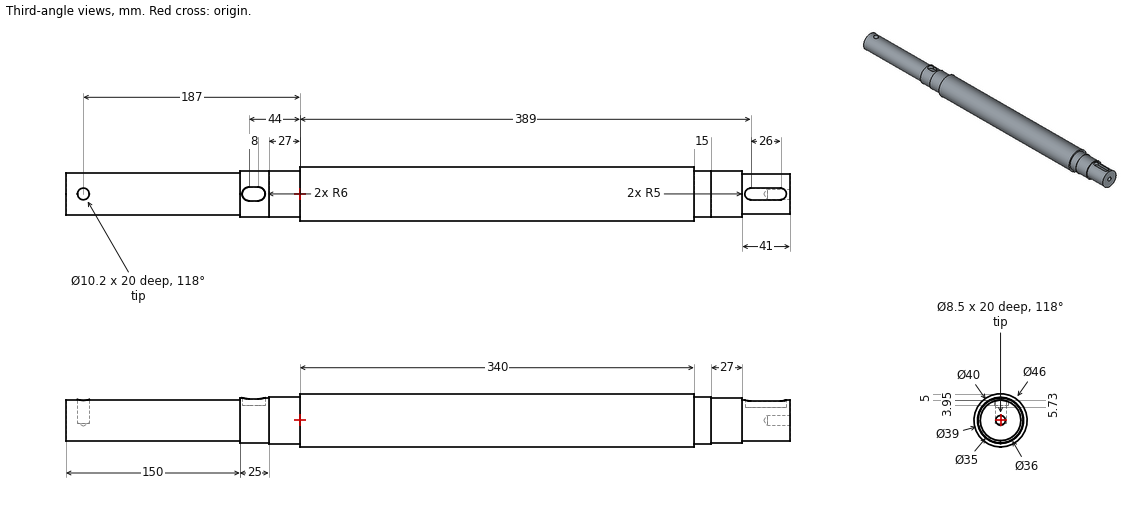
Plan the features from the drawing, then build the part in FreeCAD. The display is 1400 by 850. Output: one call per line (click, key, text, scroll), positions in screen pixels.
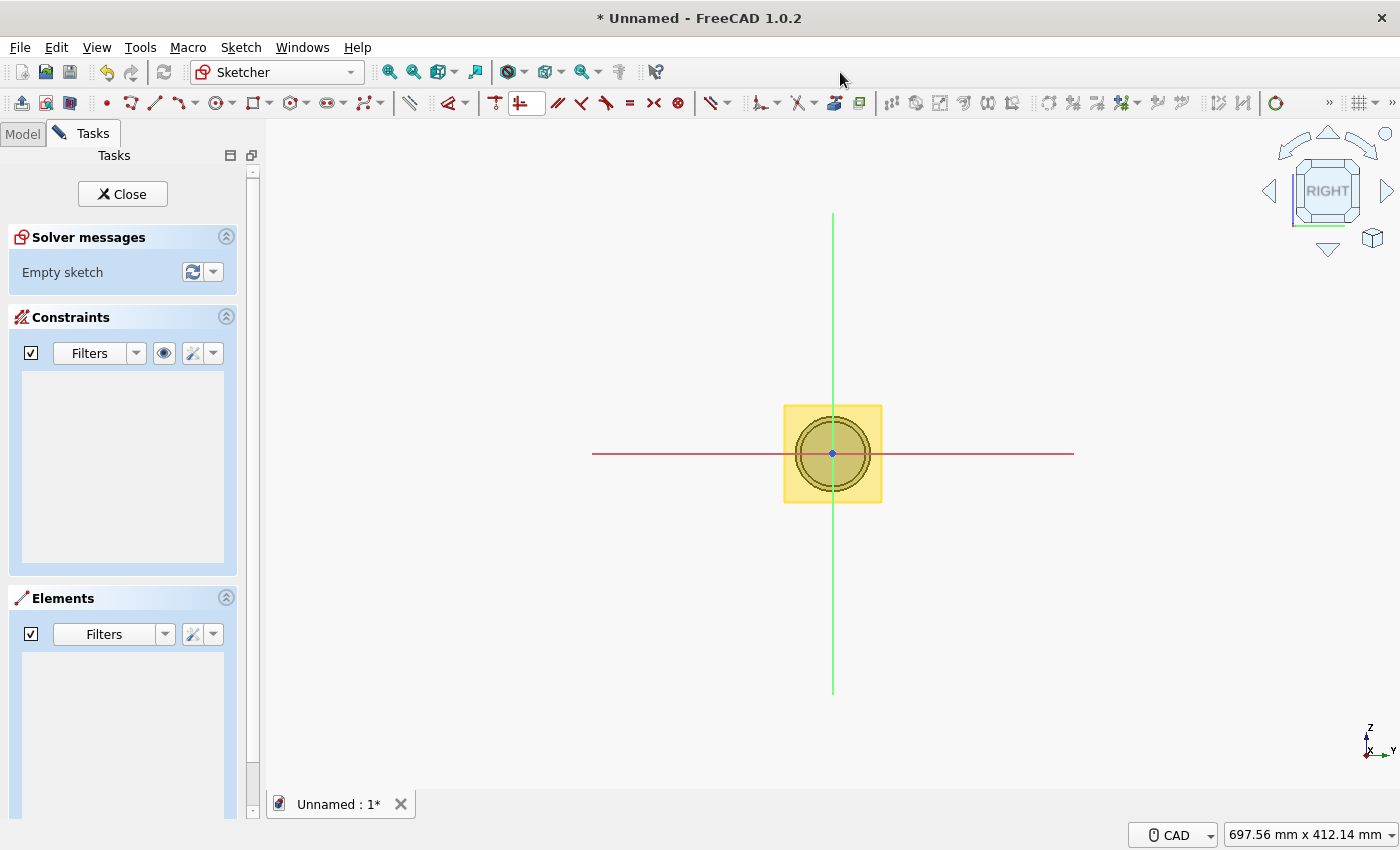
scroll(844, 454, up, 10)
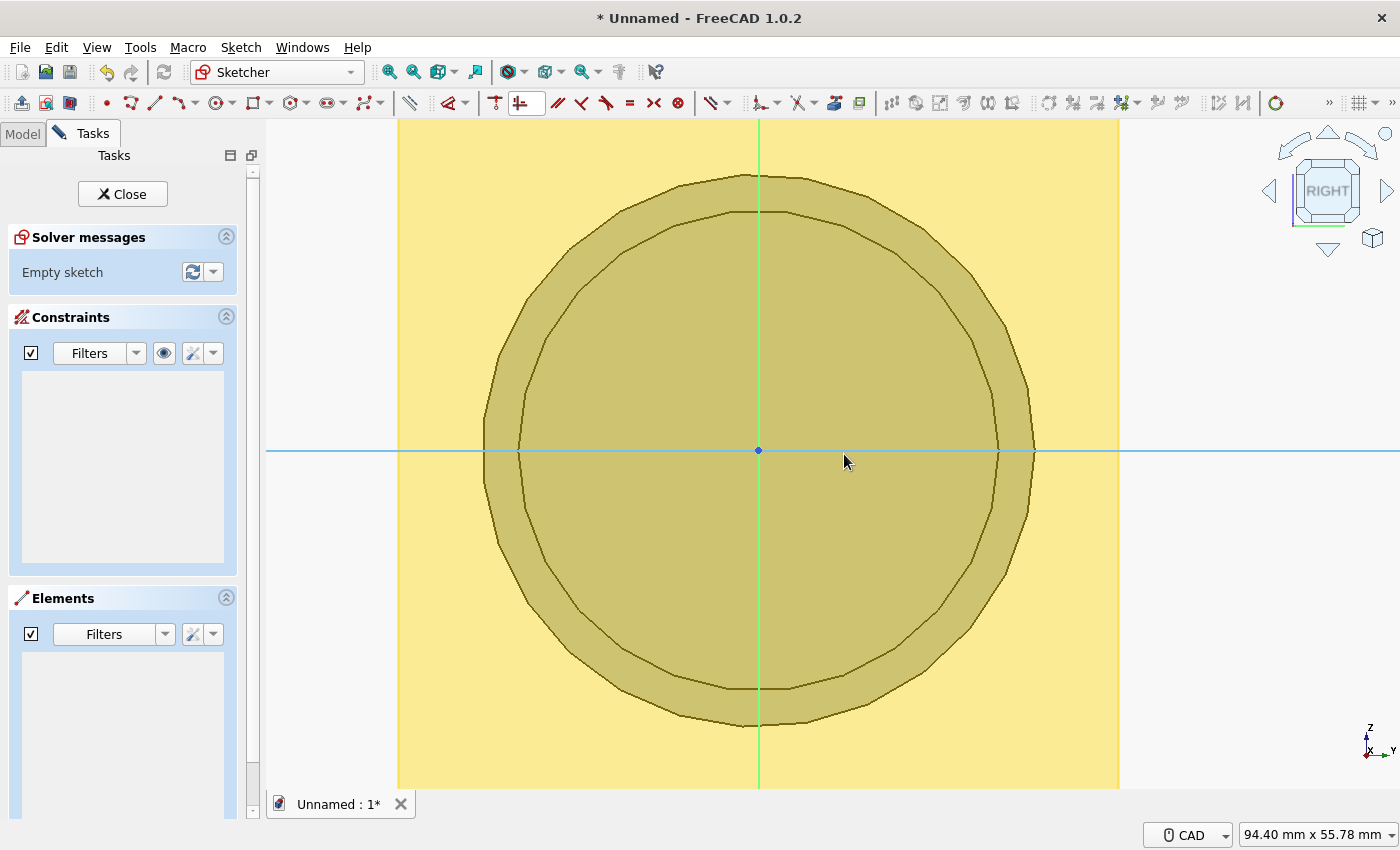
click(216, 104)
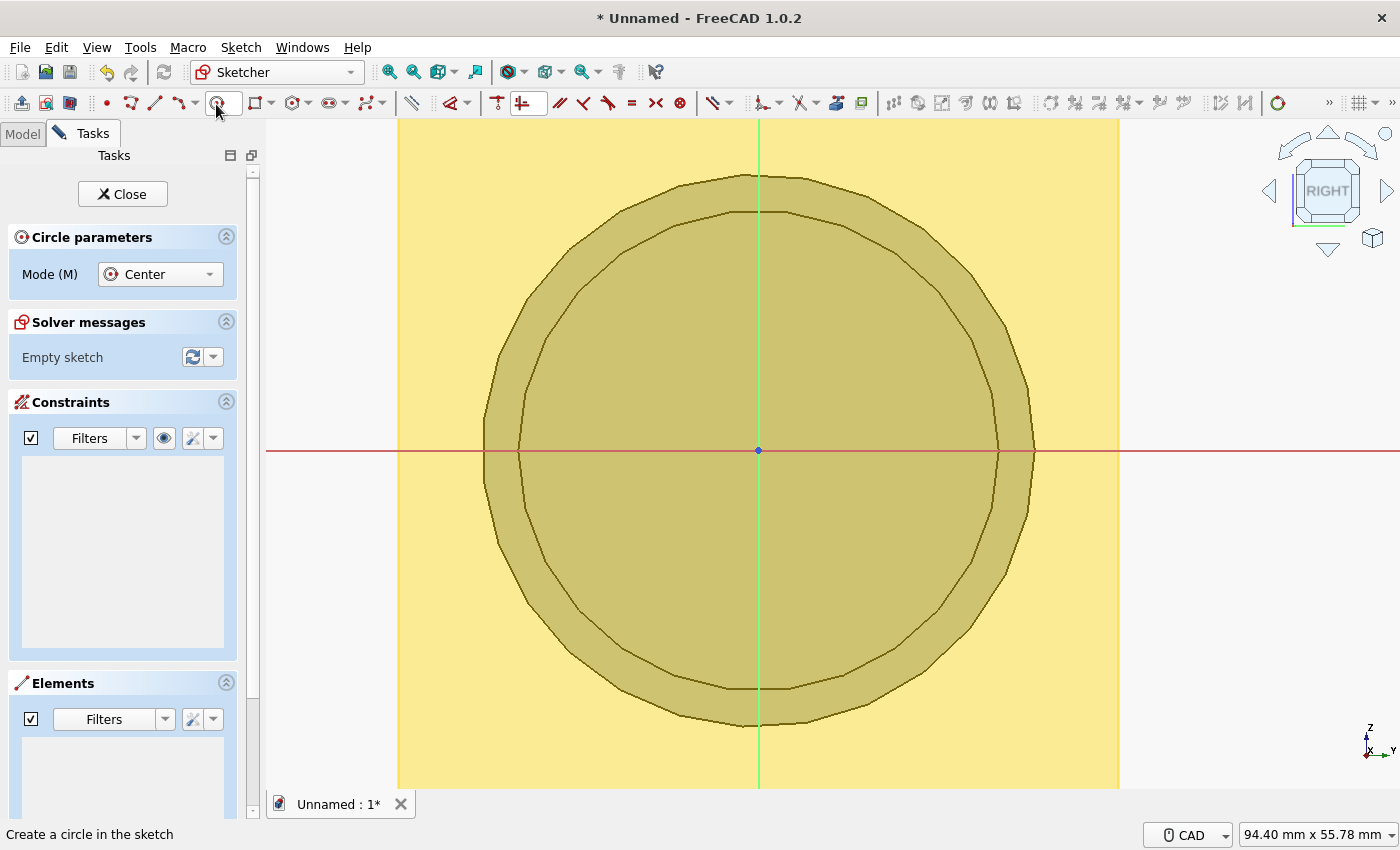
click(759, 451)
click(924, 285)
key(Escape)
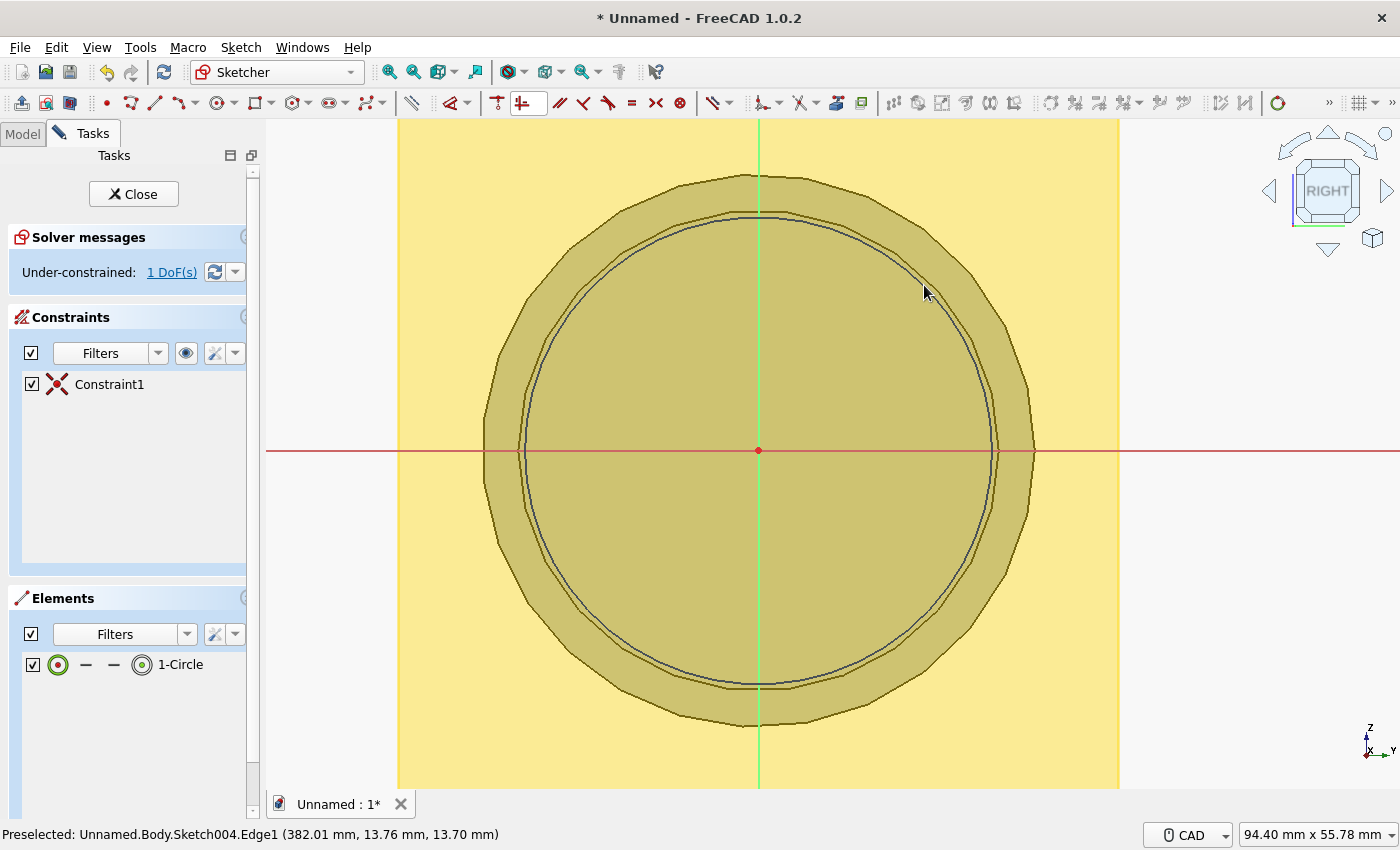
key(d)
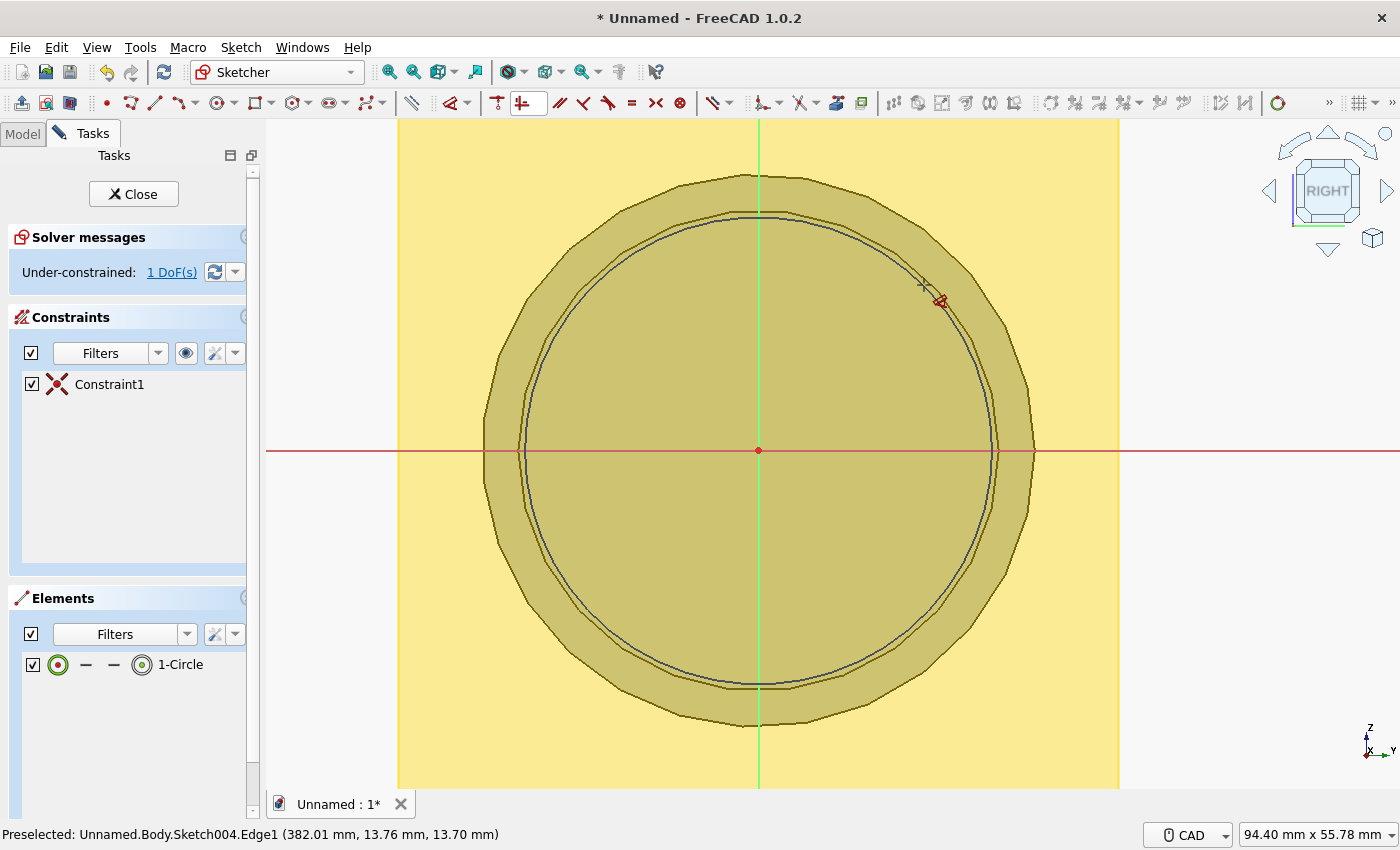
click(923, 285)
click(946, 262)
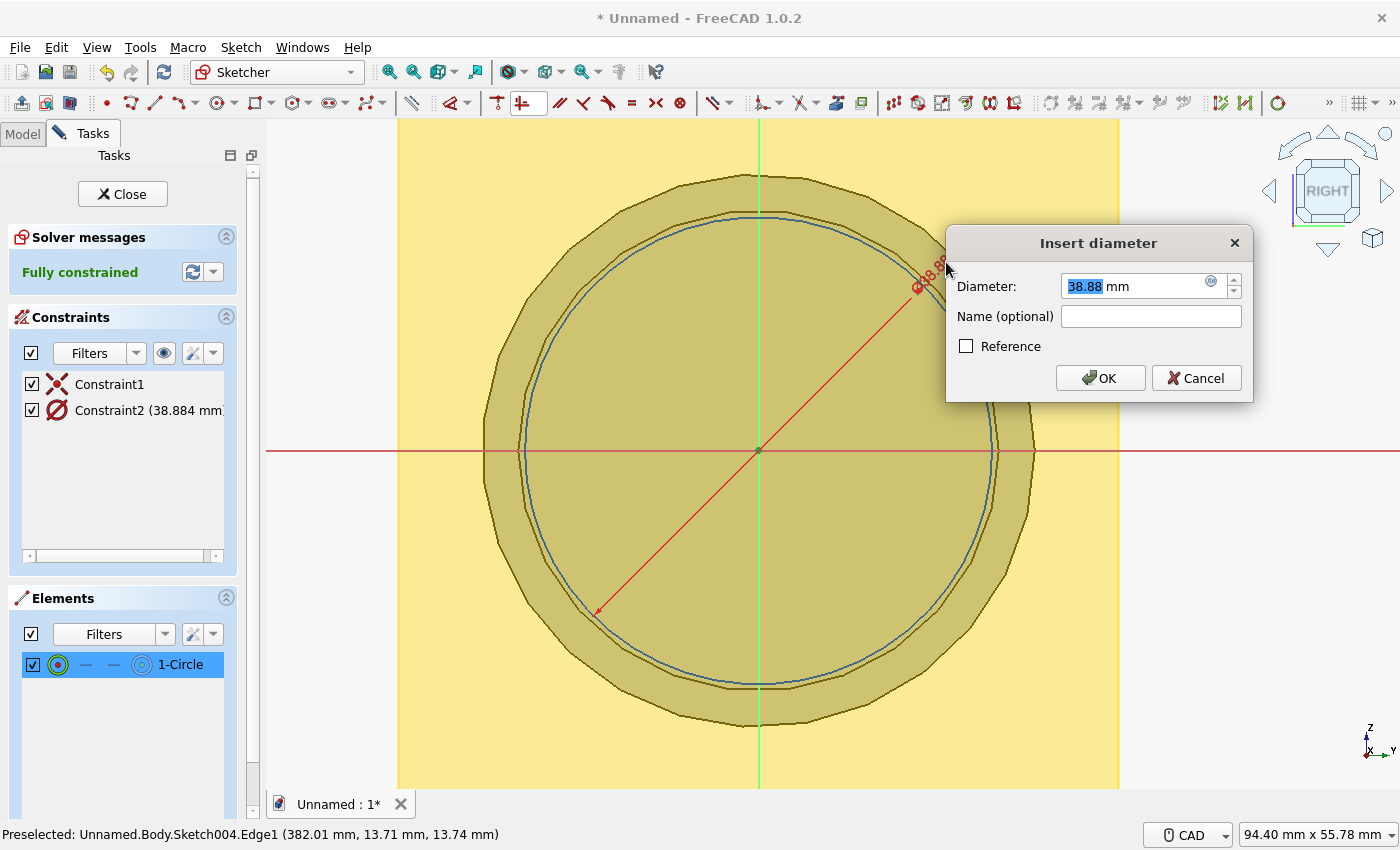
text(39)
key(Return)
key(Escape)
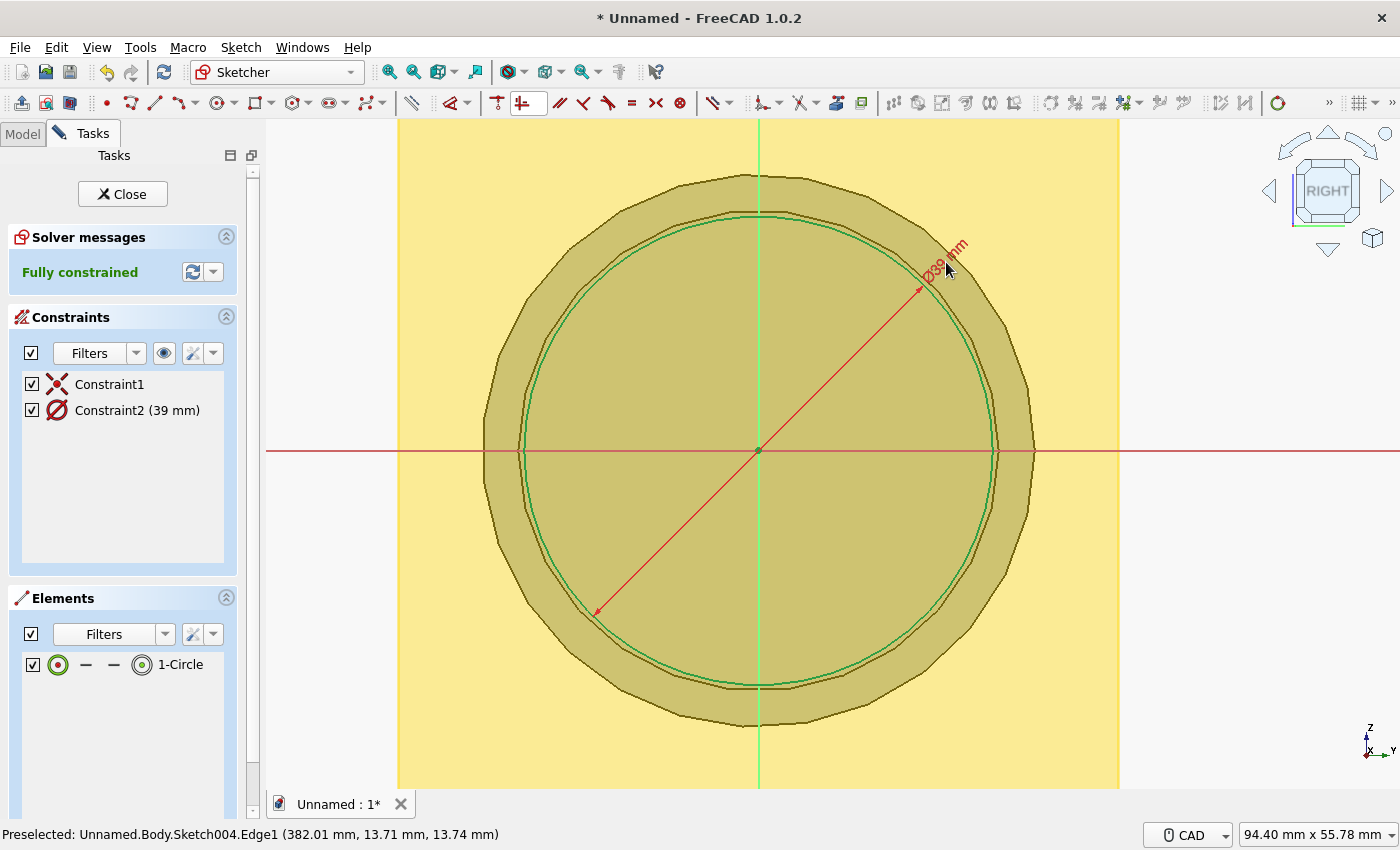
click(123, 194)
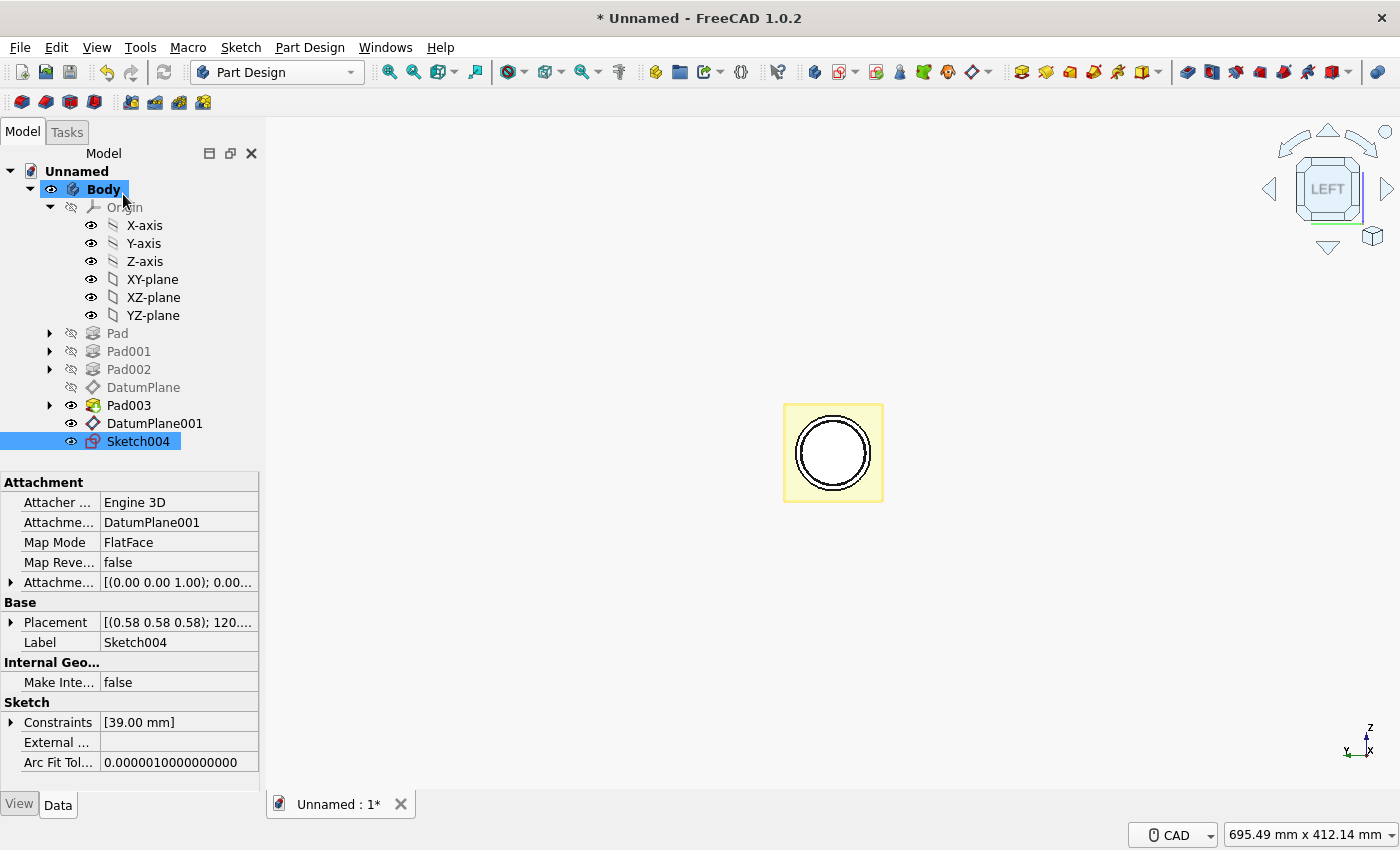
click(1022, 72)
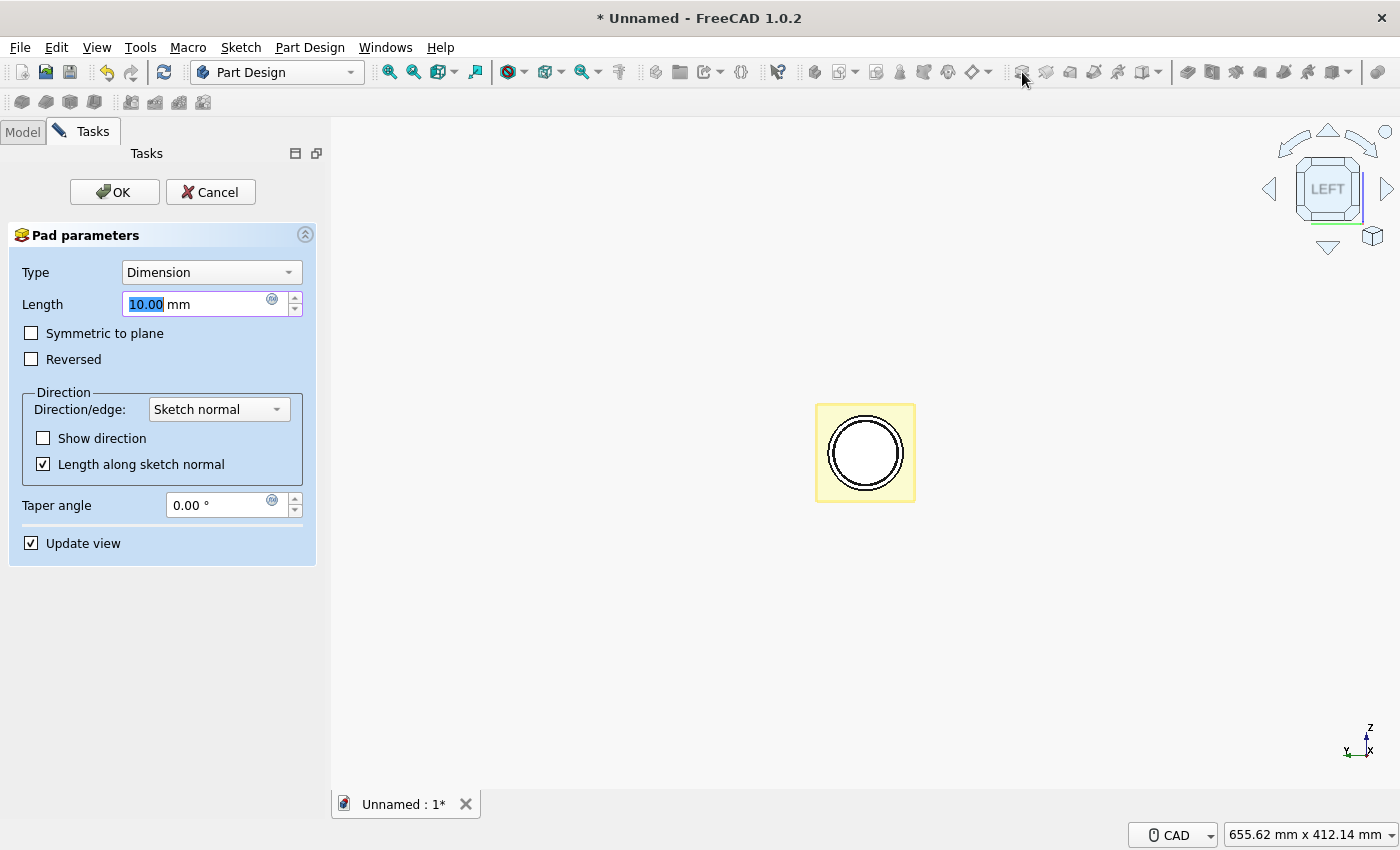
text(27)
key(Tab)